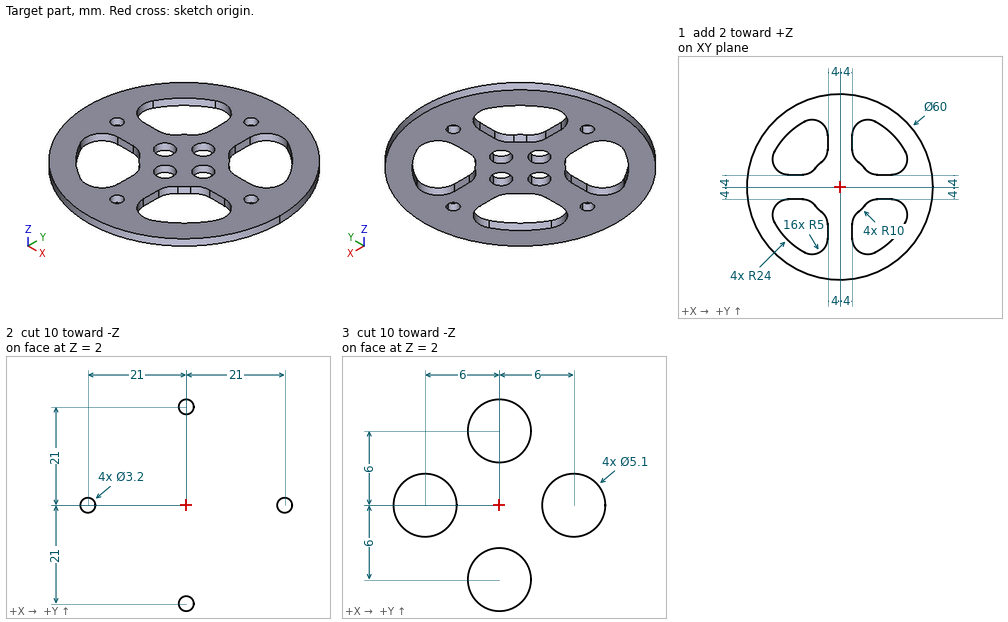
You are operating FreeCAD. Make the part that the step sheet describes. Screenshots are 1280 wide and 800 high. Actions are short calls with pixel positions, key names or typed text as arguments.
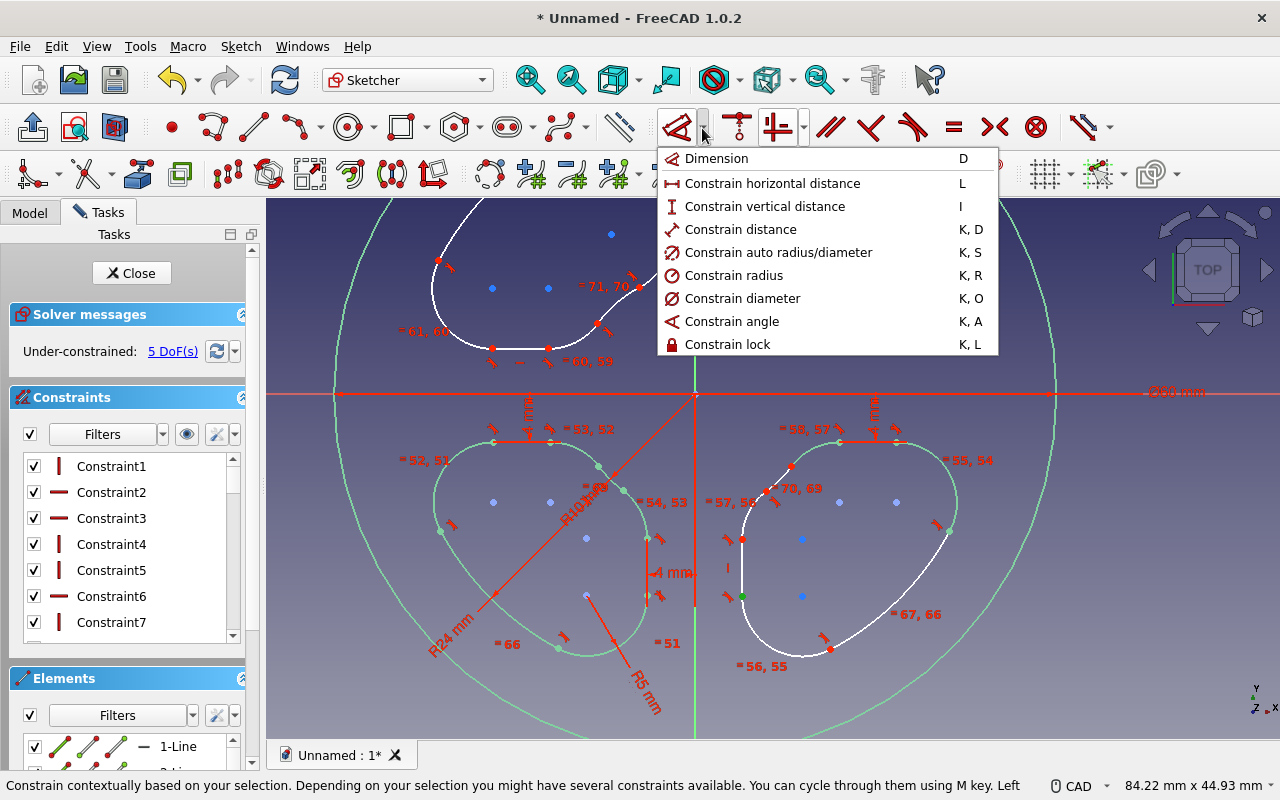
click(828, 184)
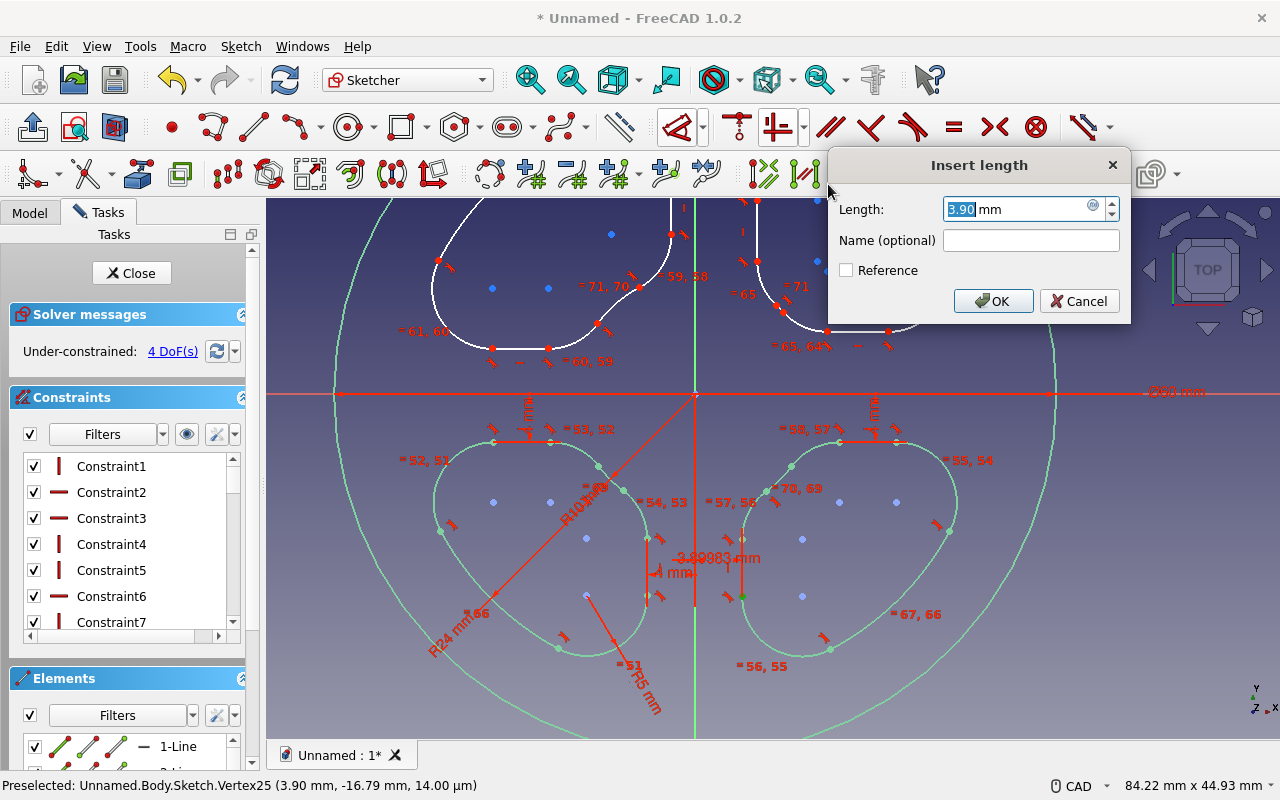
text(4)
key(Return)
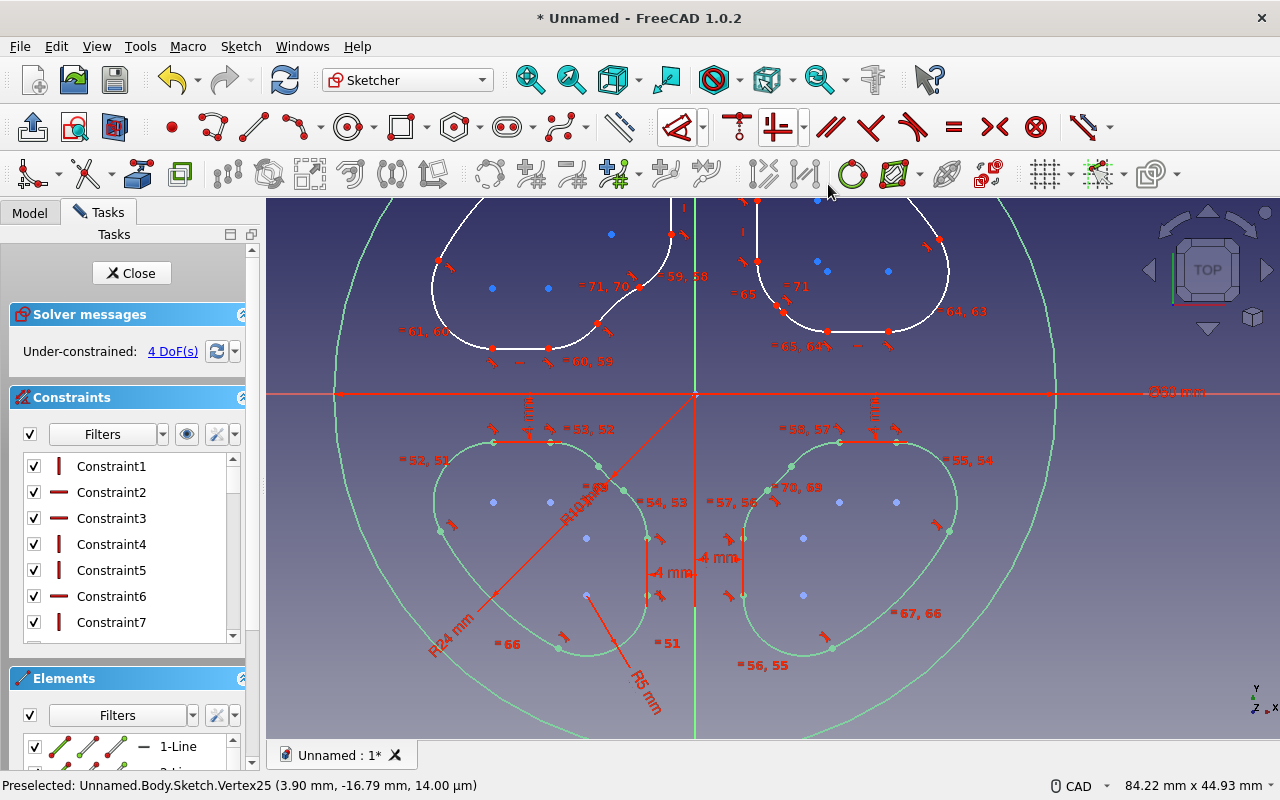
scroll(712, 529, down, 4)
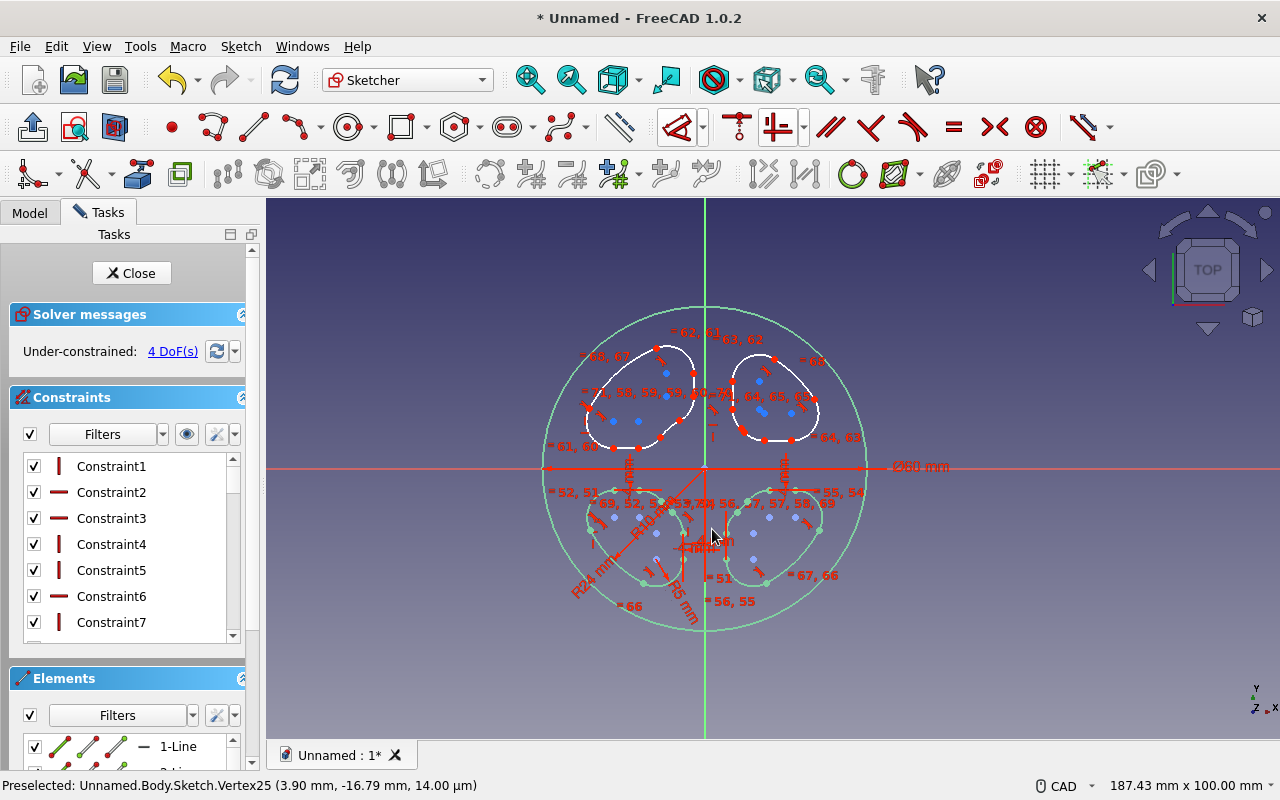
scroll(694, 373, up, 4)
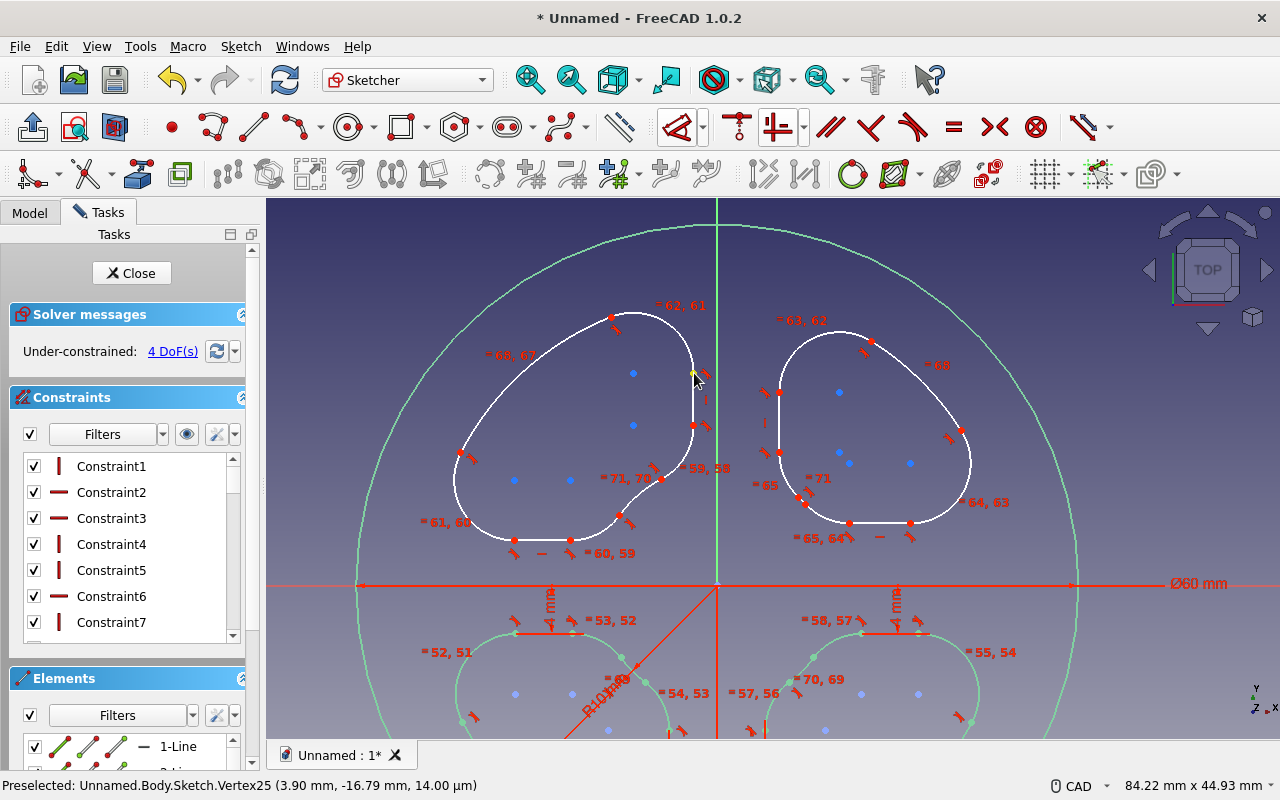
click(693, 373)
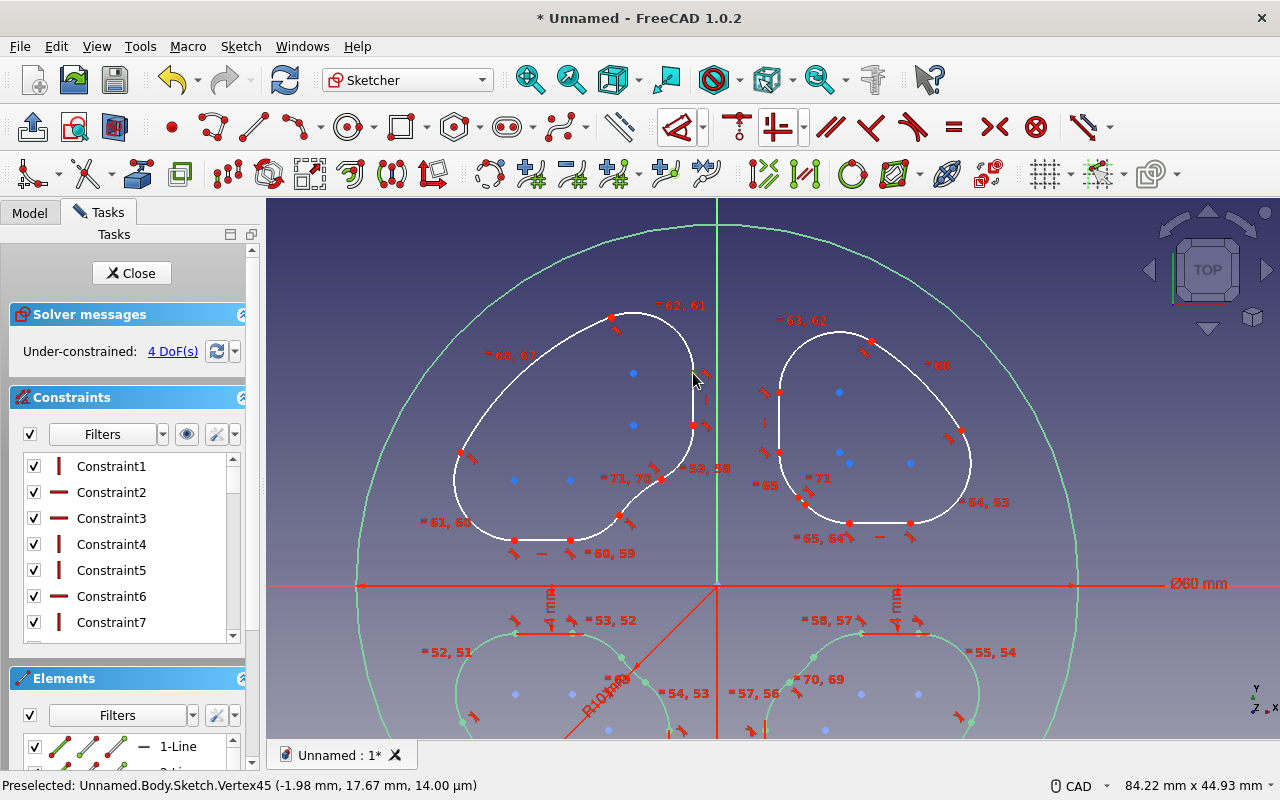
click(702, 128)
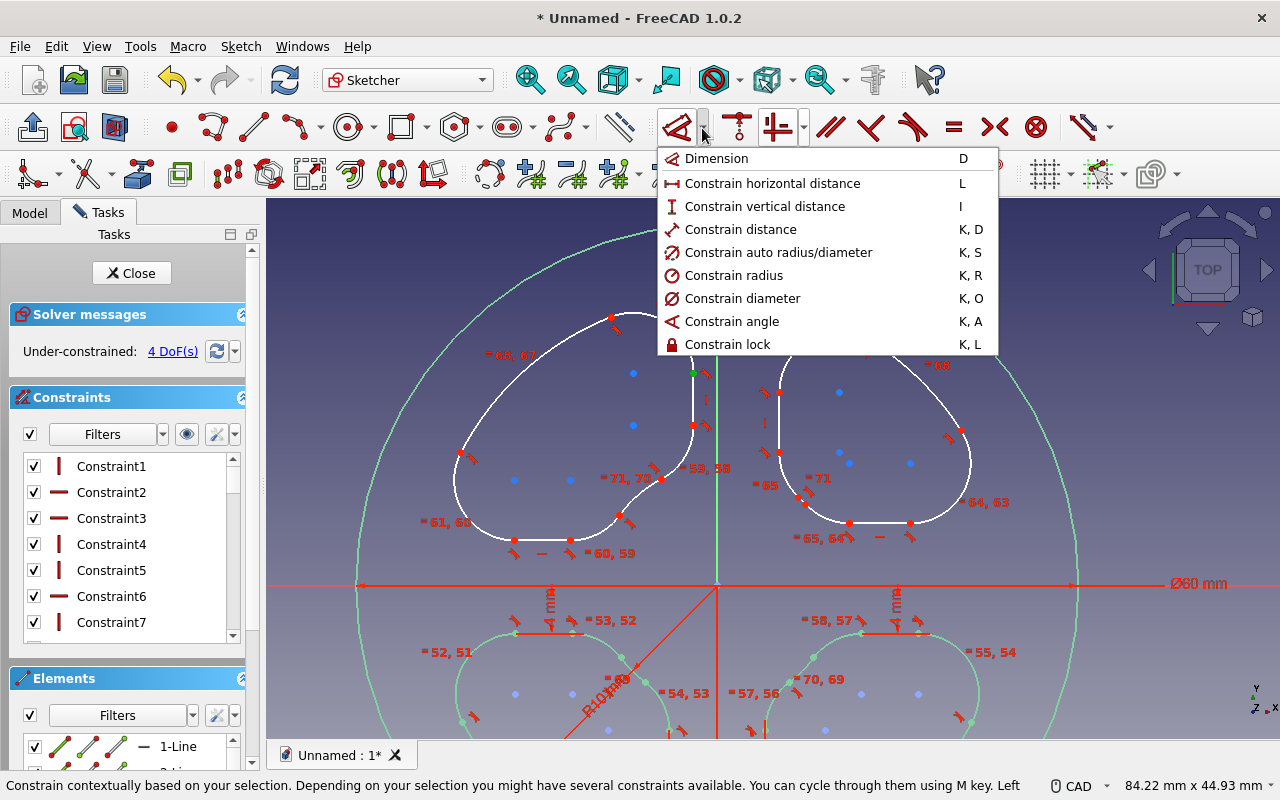
click(828, 184)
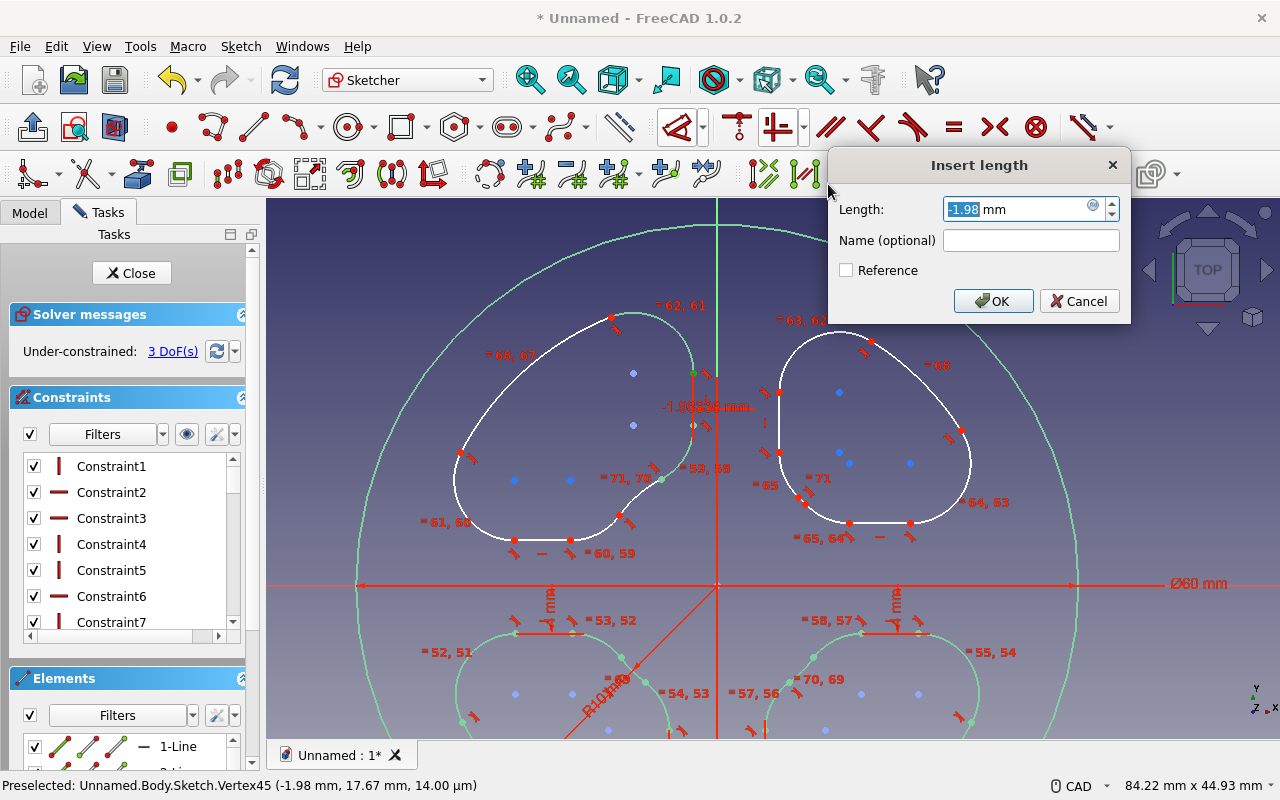
text(-4)
key(Return)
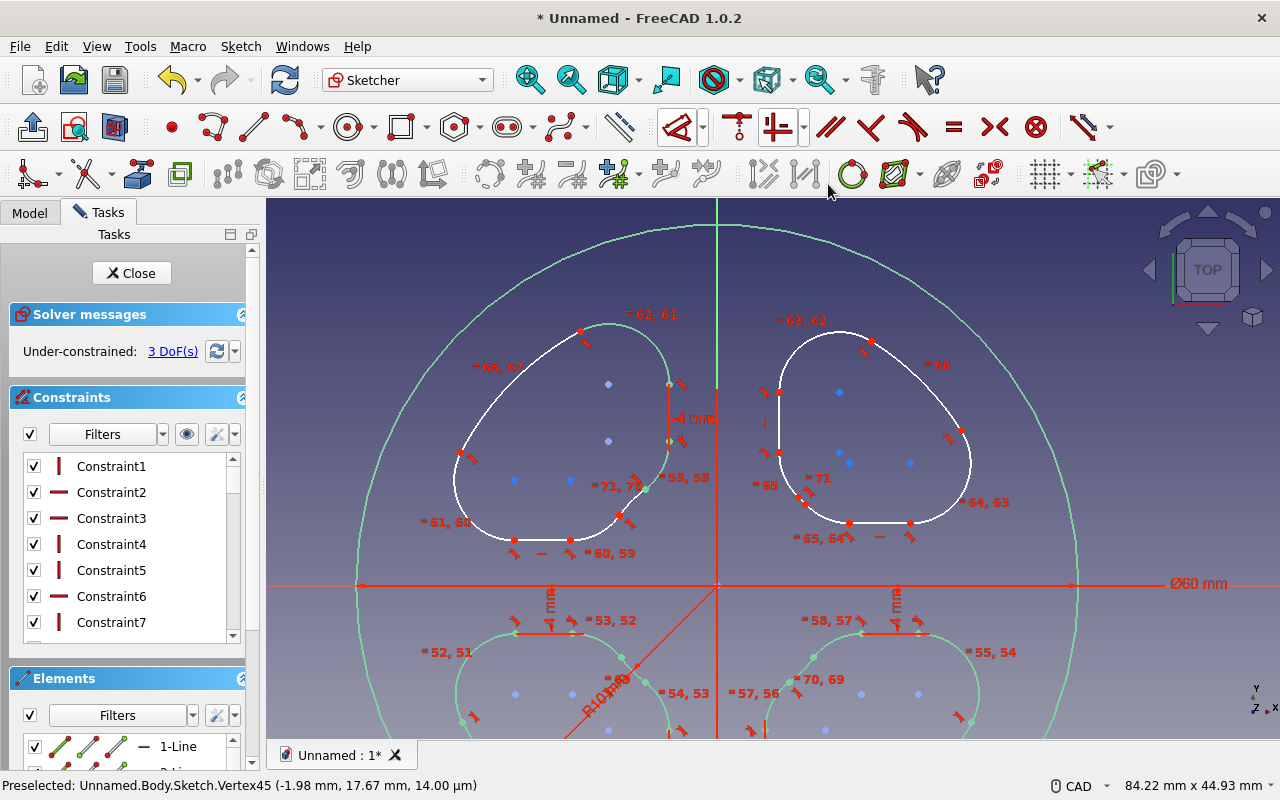
click(571, 540)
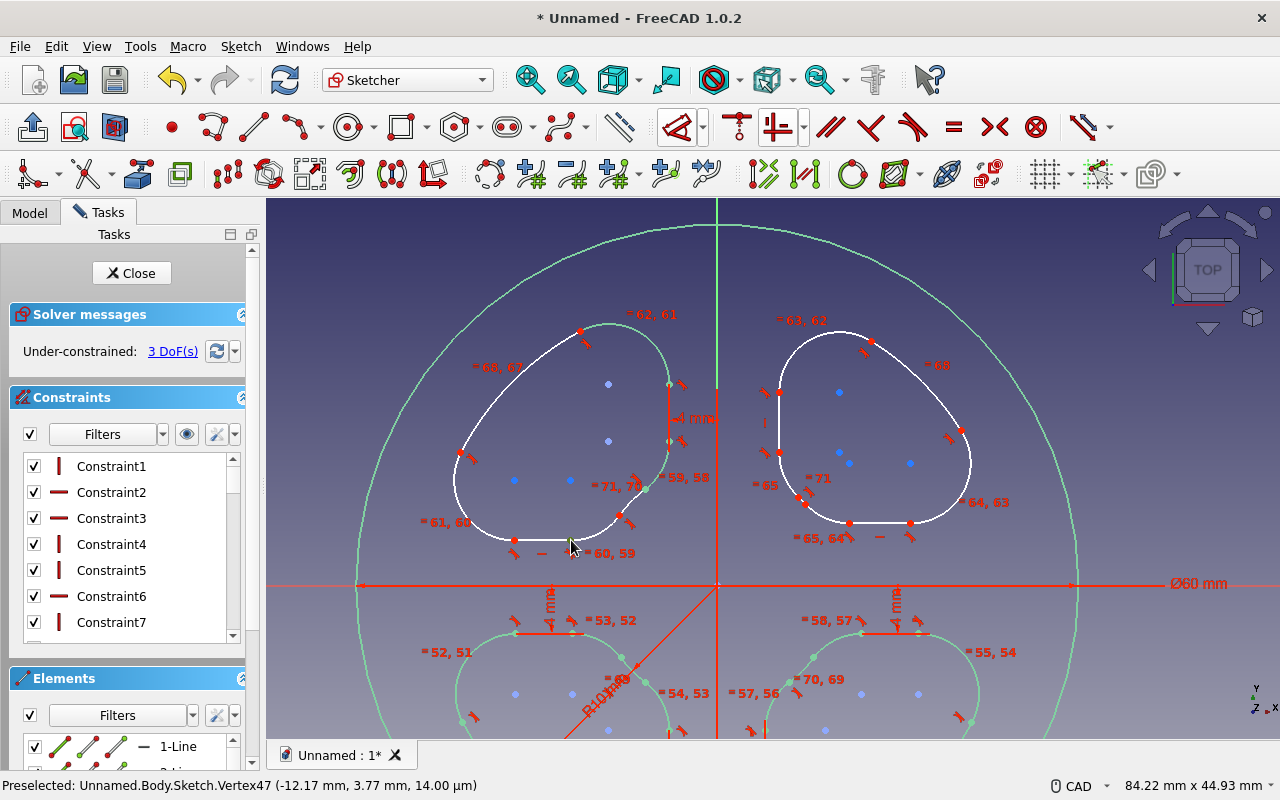
key(i)